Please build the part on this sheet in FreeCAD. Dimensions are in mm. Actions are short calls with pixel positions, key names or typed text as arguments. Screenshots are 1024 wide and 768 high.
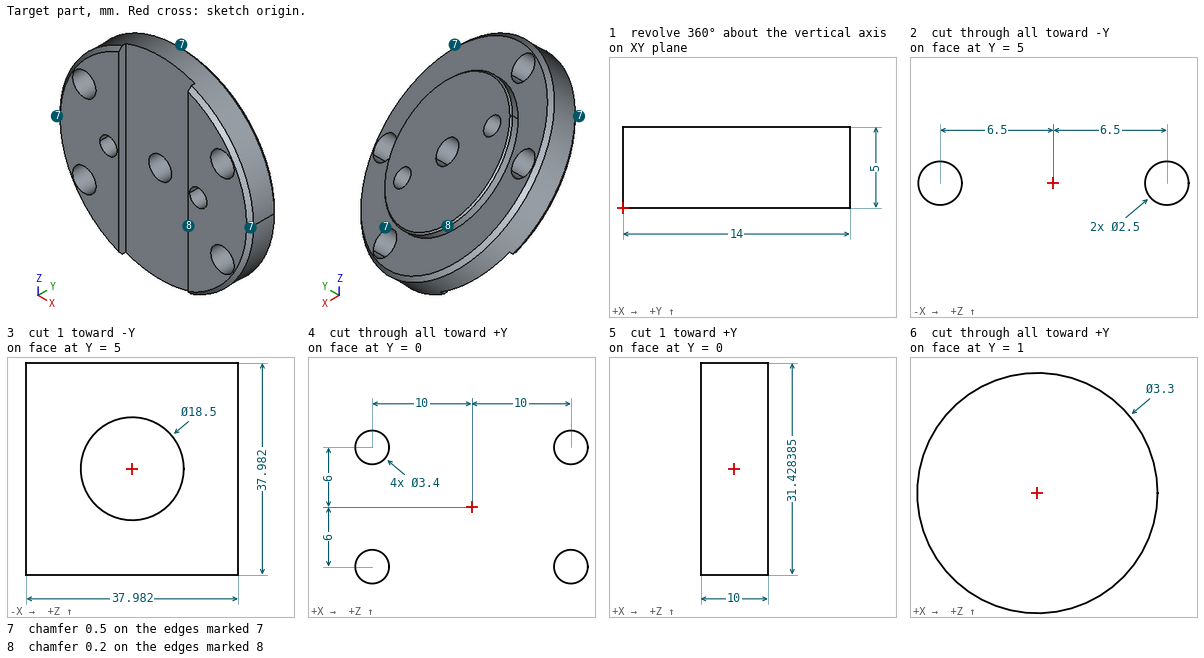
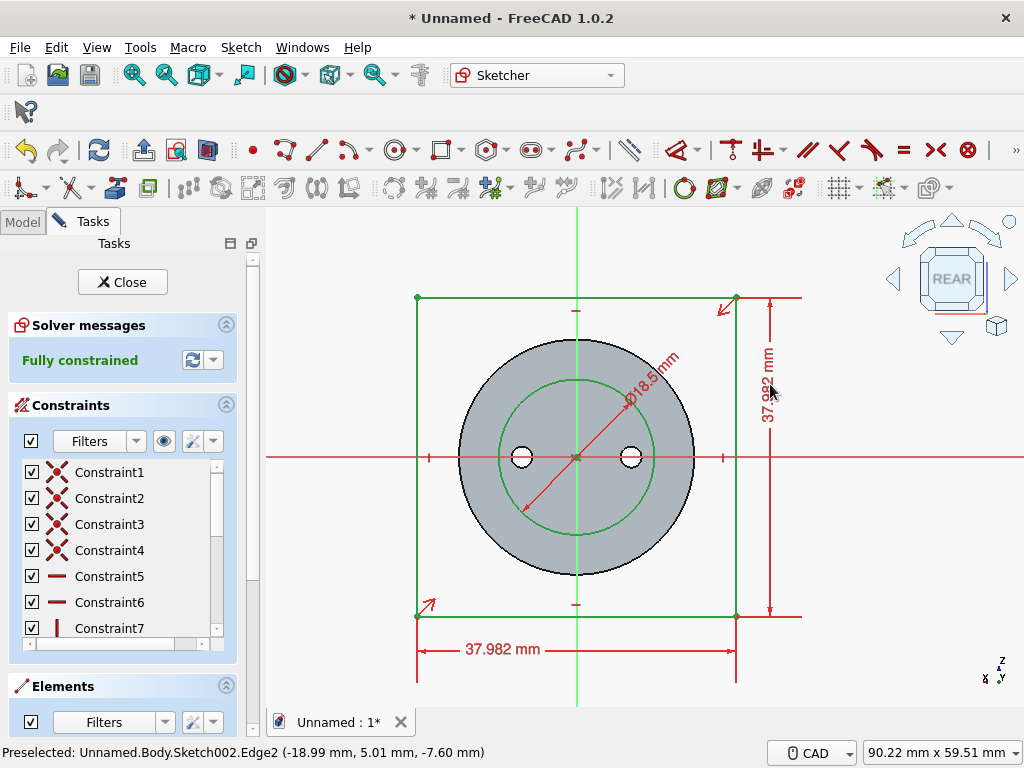
click(123, 282)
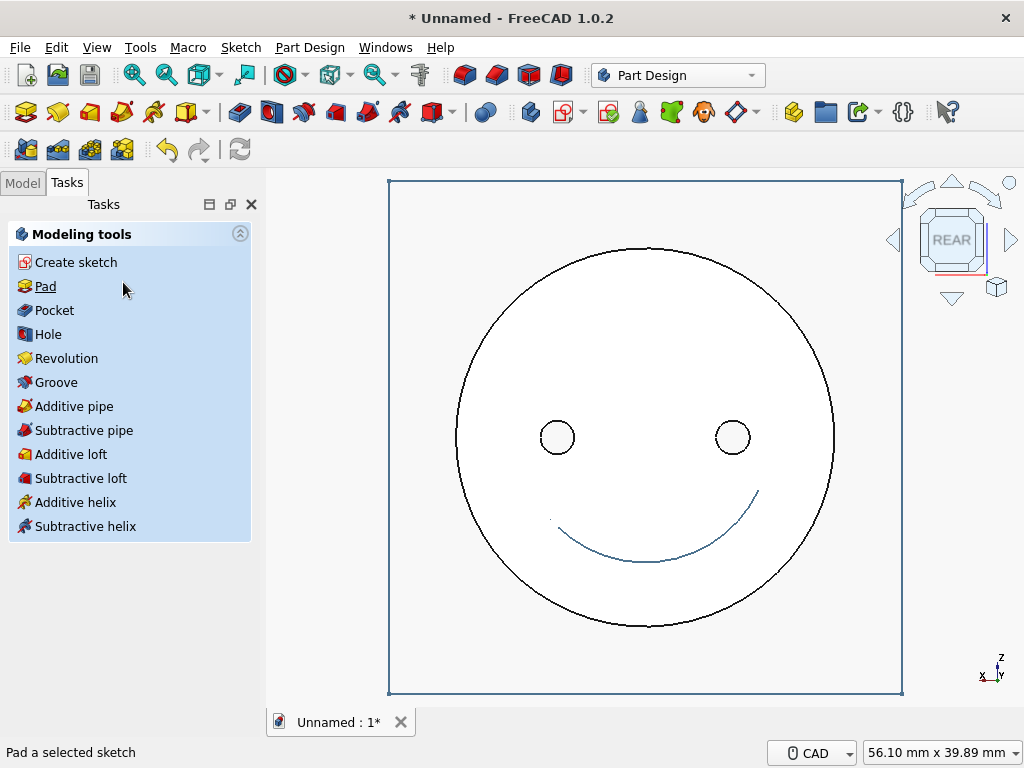
click(240, 112)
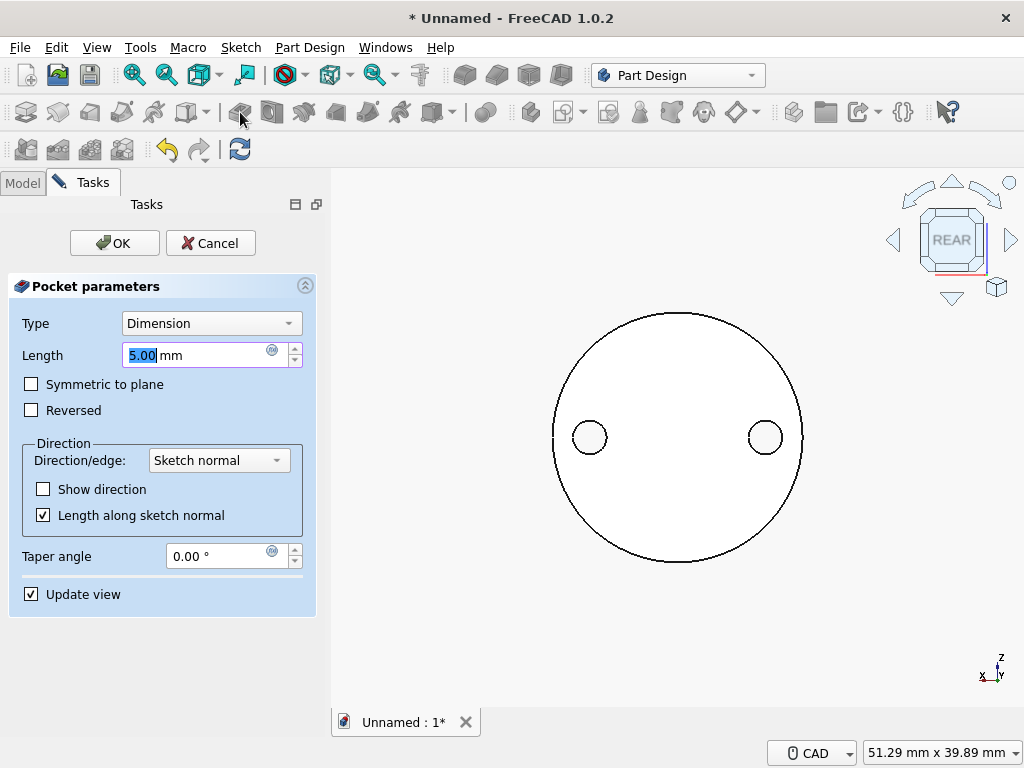
text(1)
key(Tab)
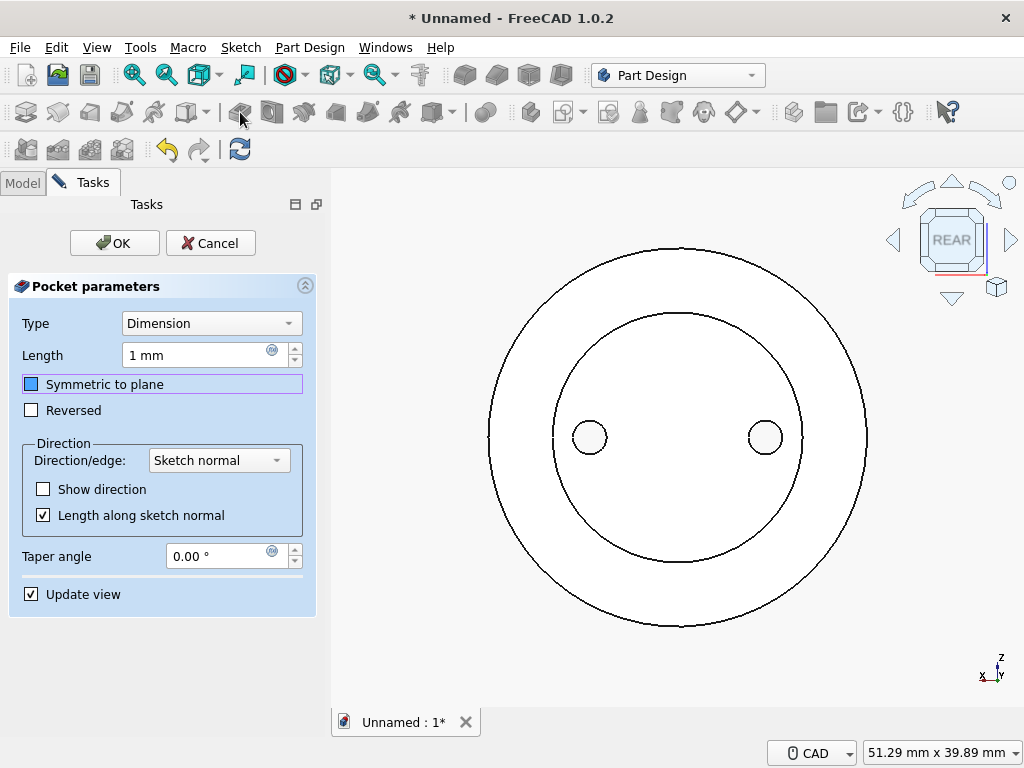
click(115, 243)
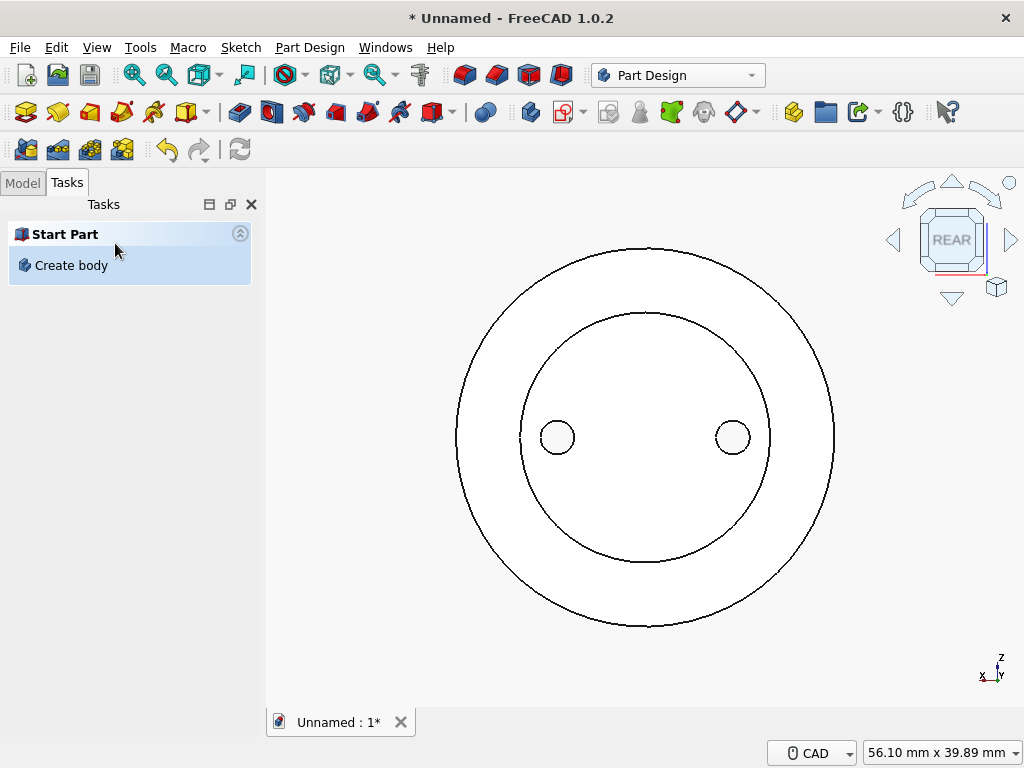
key(0)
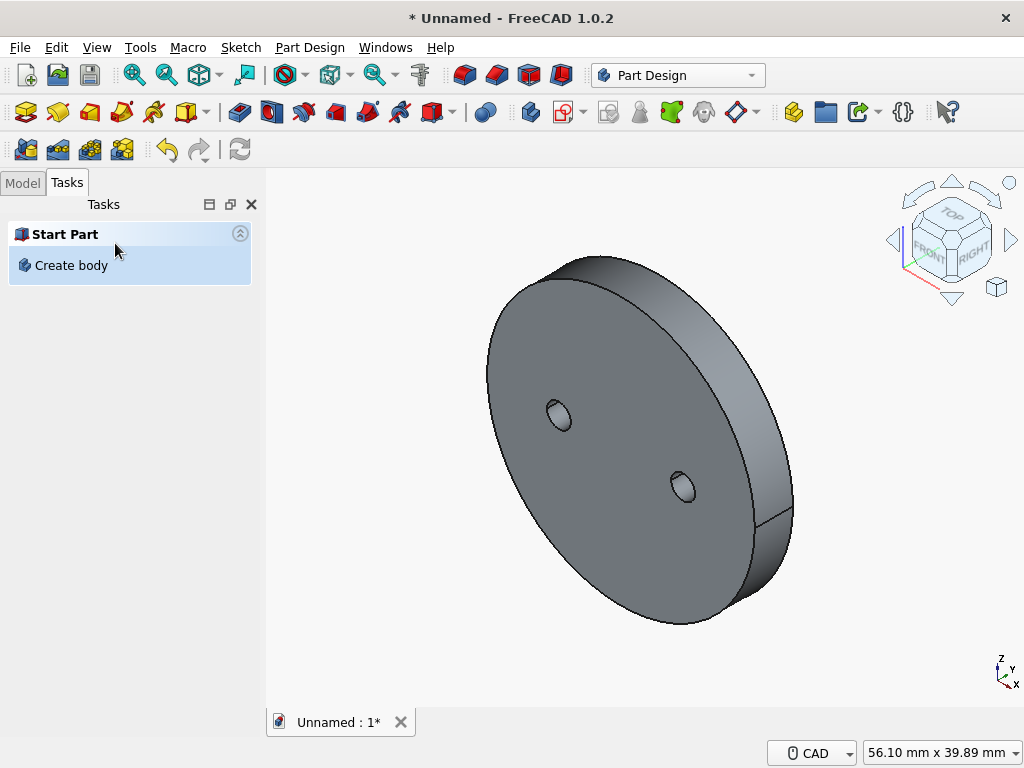
click(621, 494)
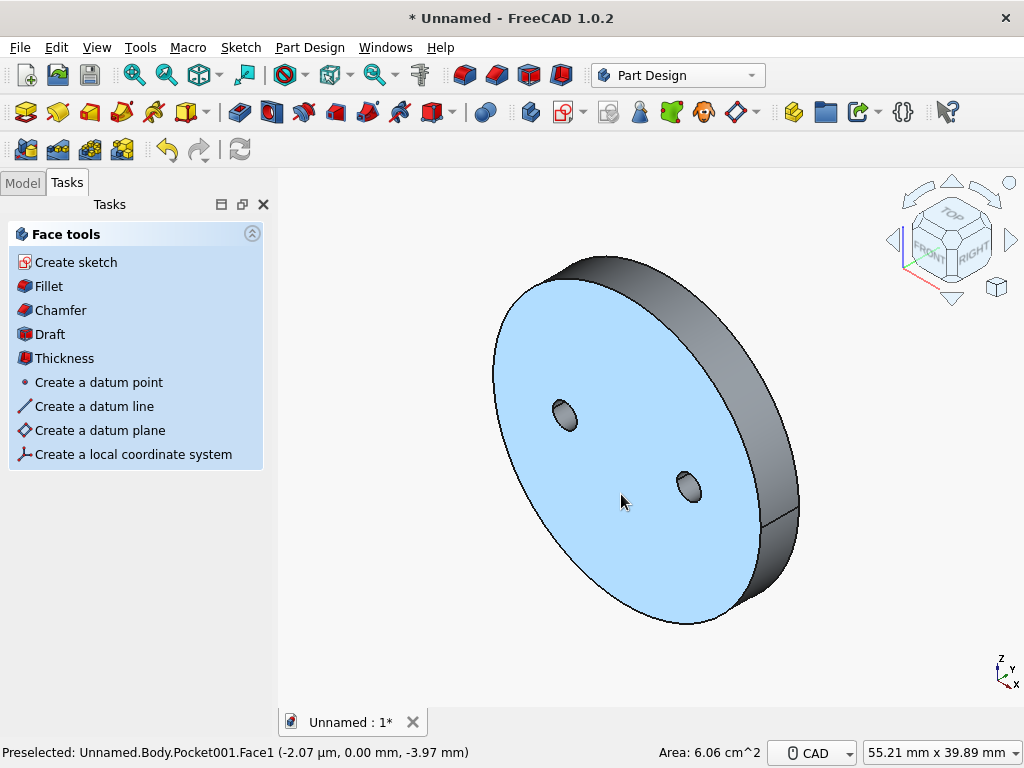
click(564, 112)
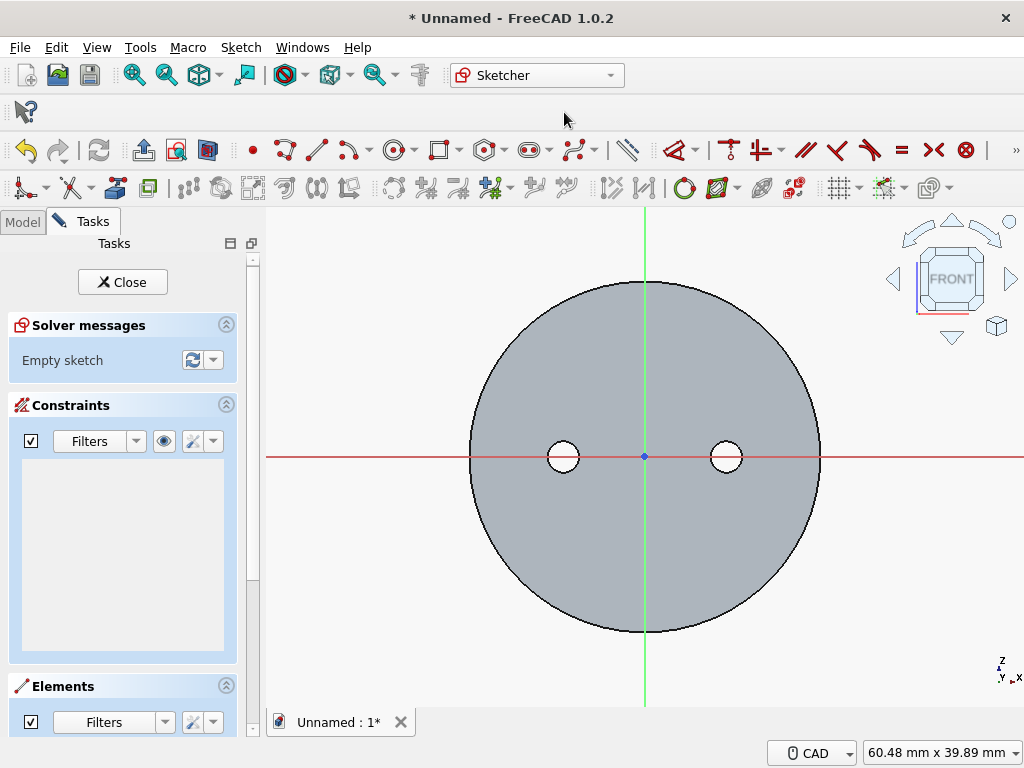
scroll(784, 457, up, 2)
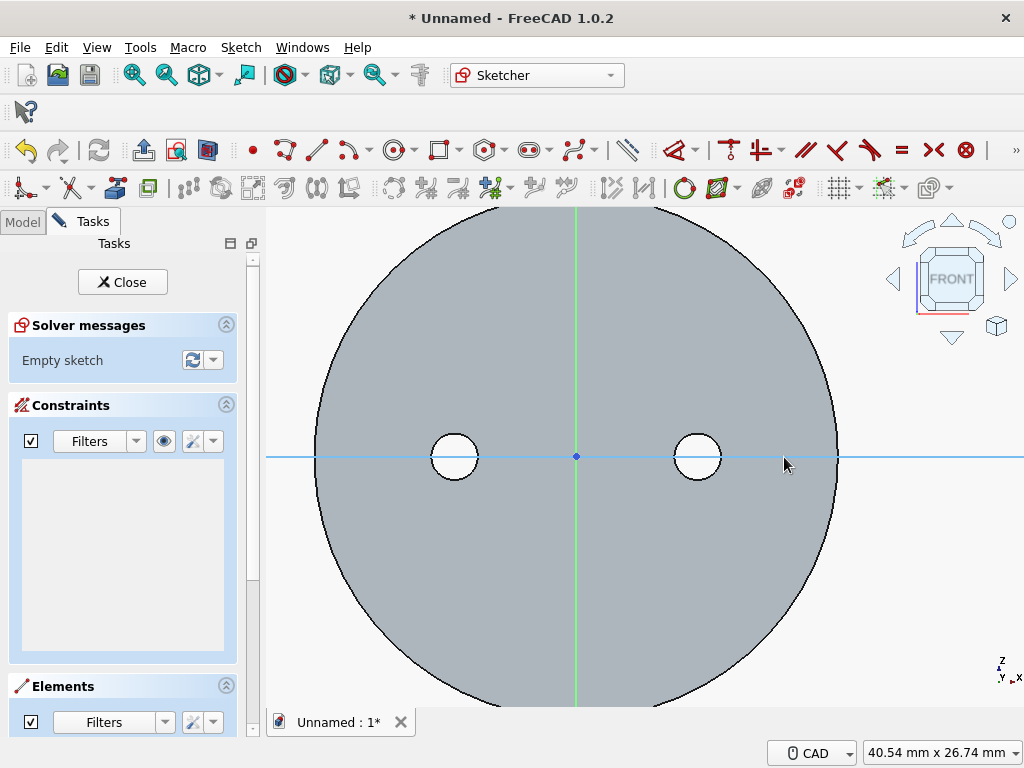
key(g)
key(c)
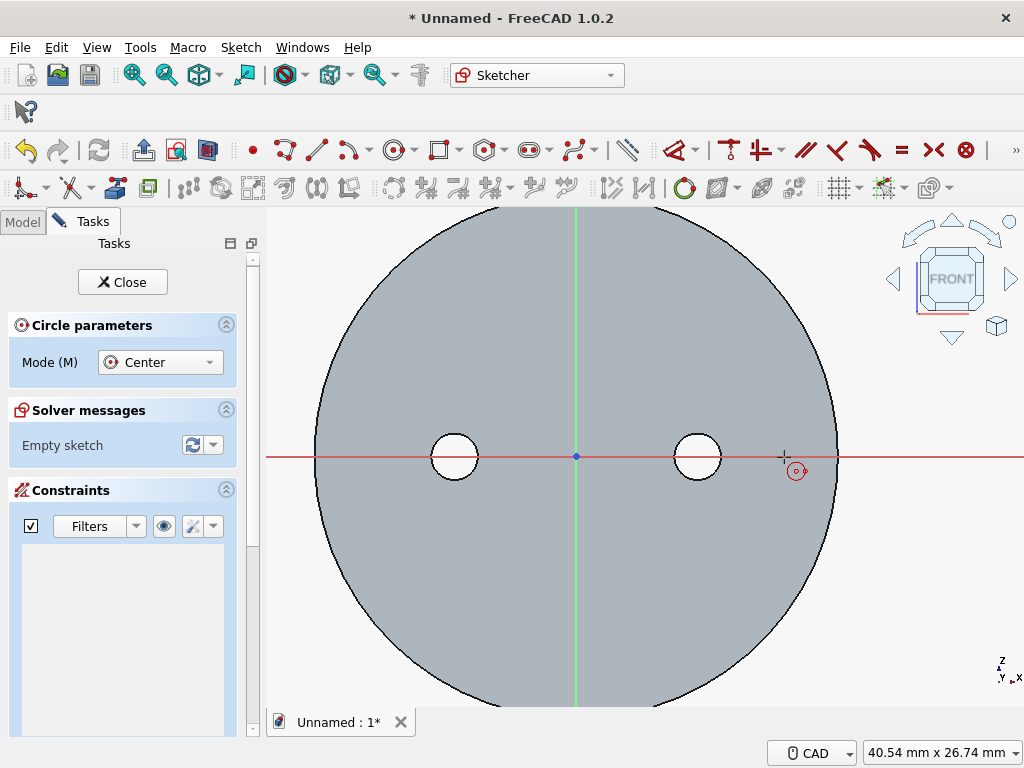
click(389, 345)
click(412, 322)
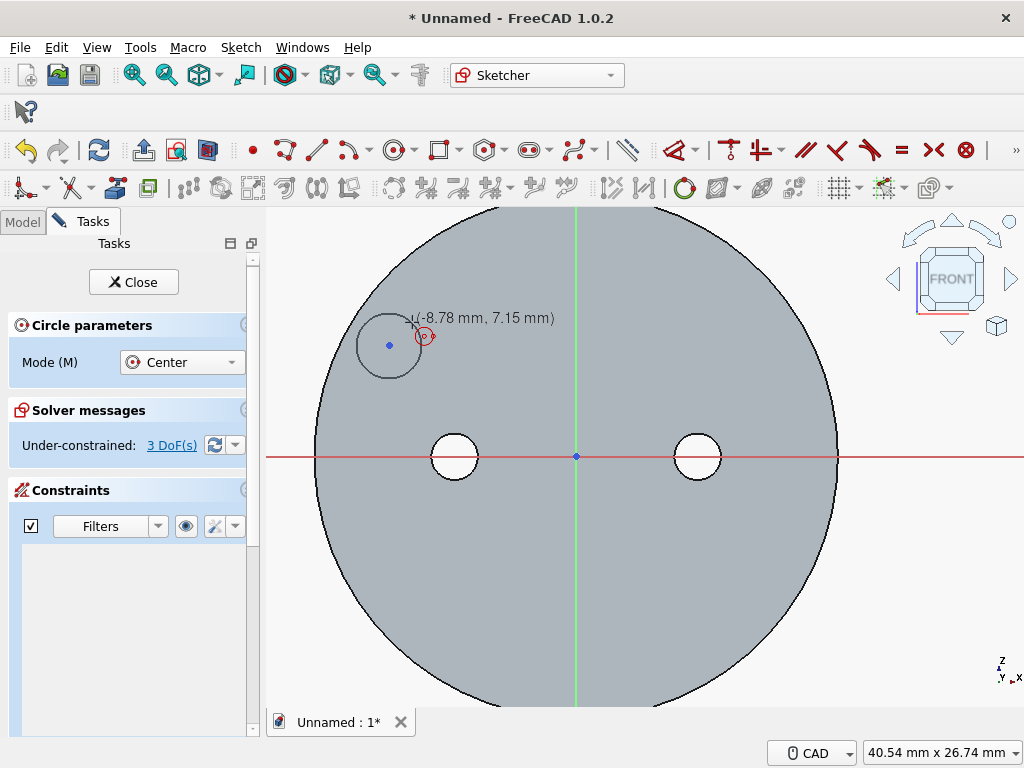
click(389, 569)
click(412, 546)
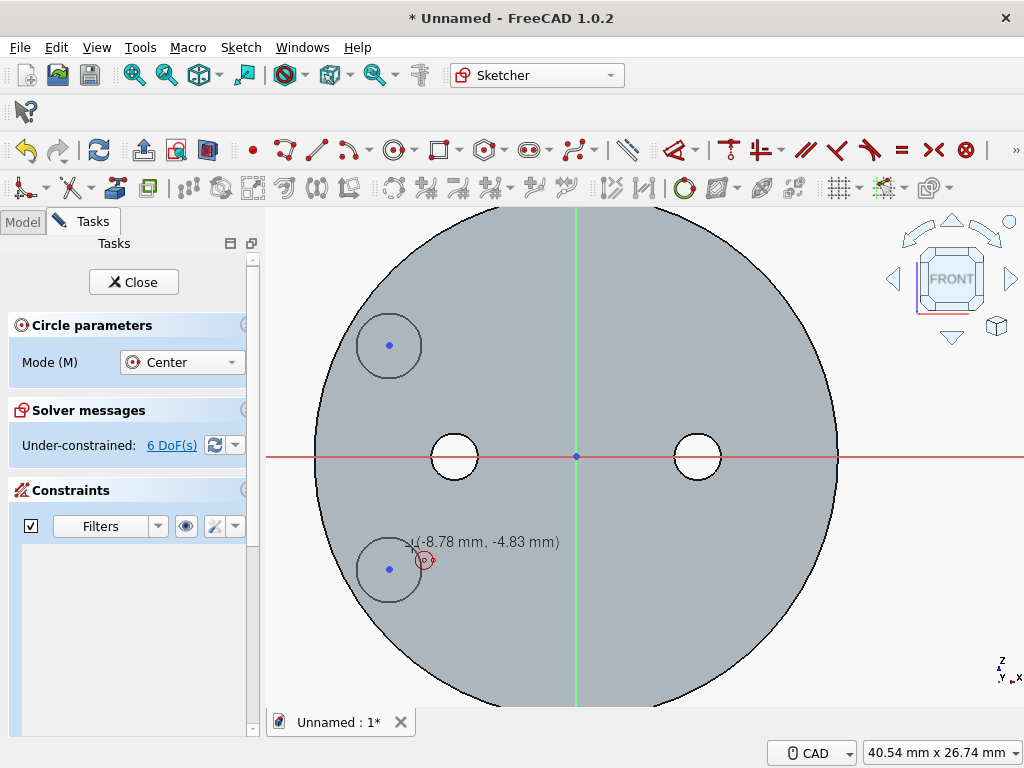
click(763, 345)
click(786, 322)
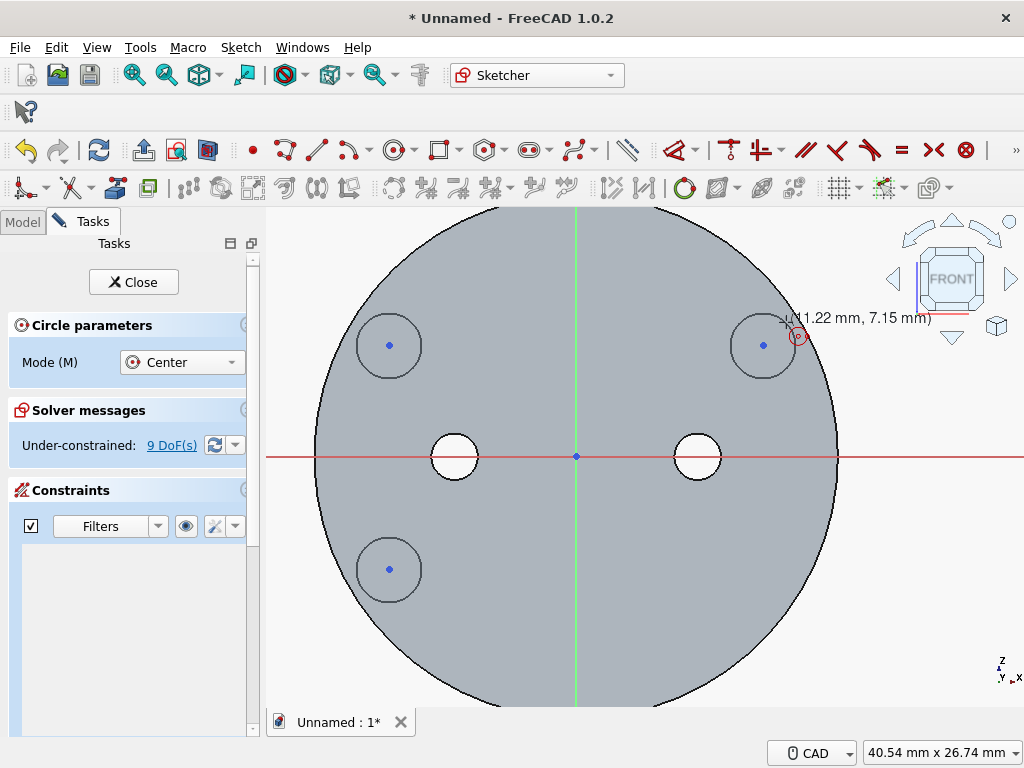
click(763, 569)
click(786, 546)
key(Escape)